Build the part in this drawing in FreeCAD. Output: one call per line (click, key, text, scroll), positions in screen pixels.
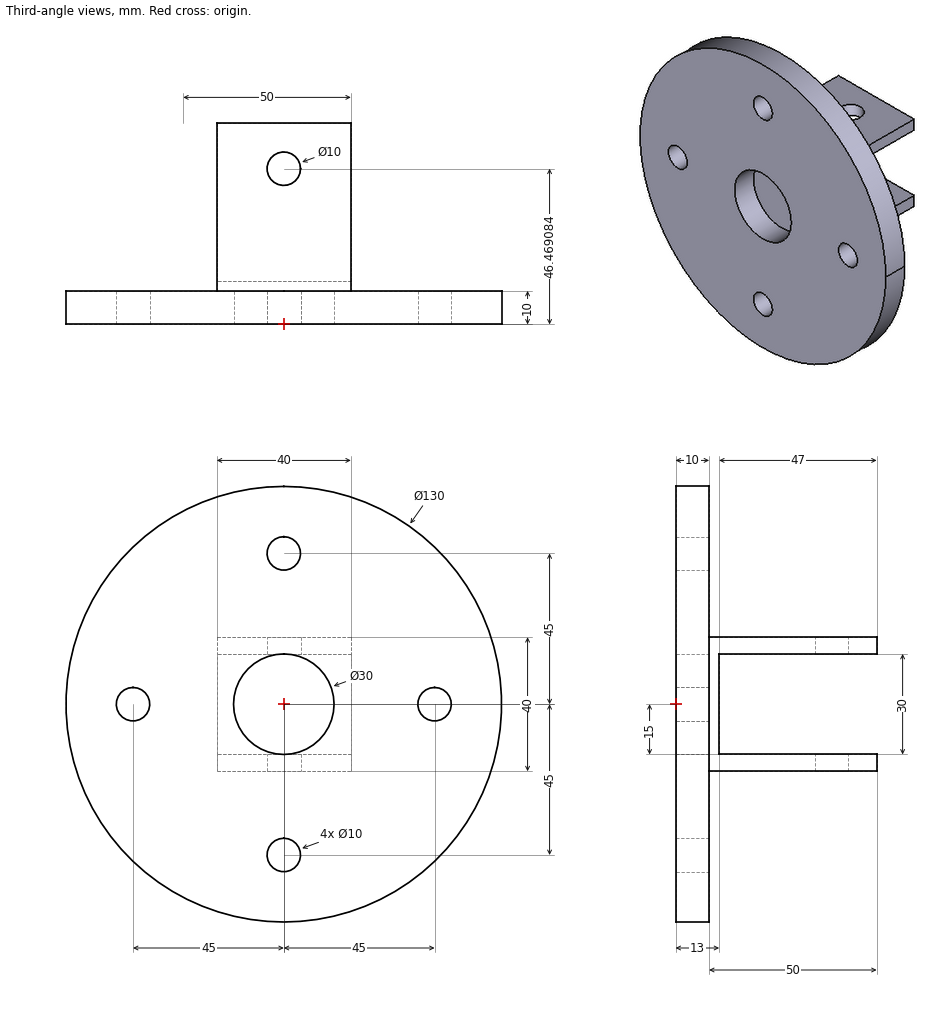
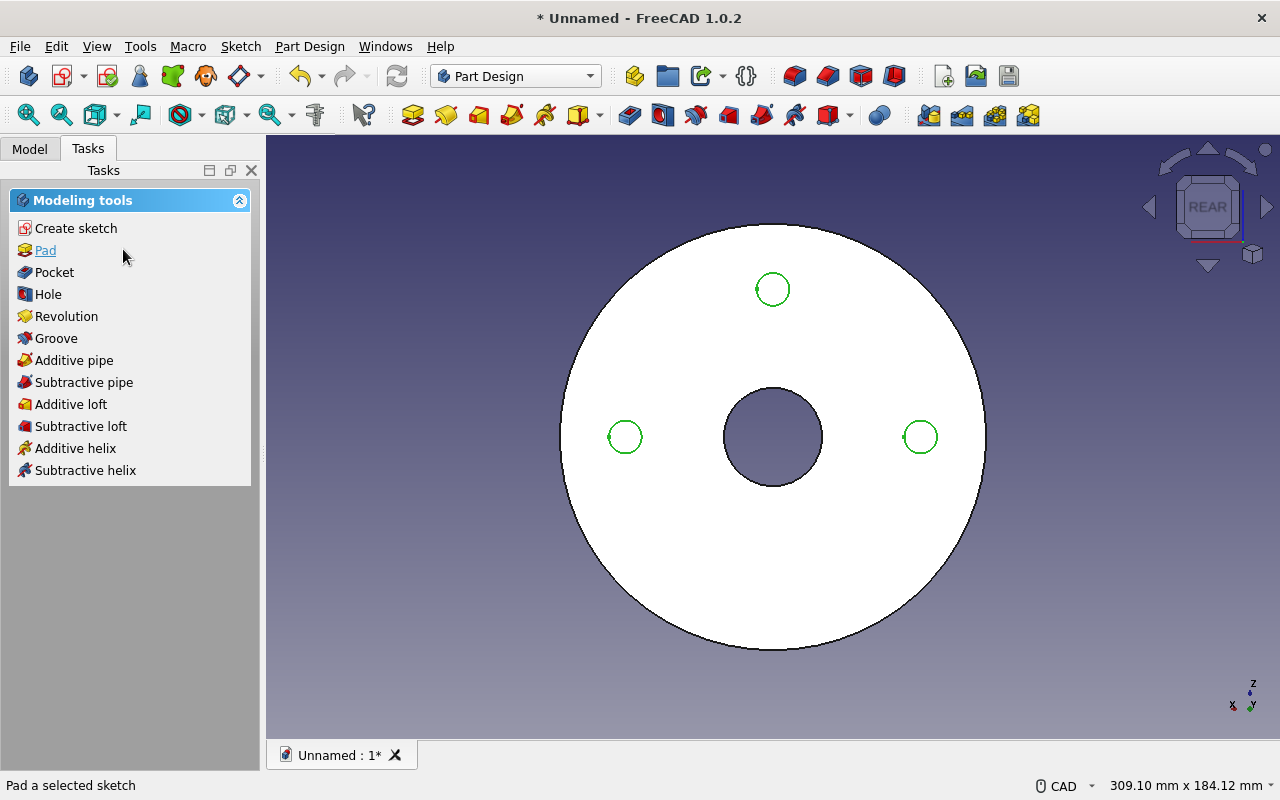
click(630, 116)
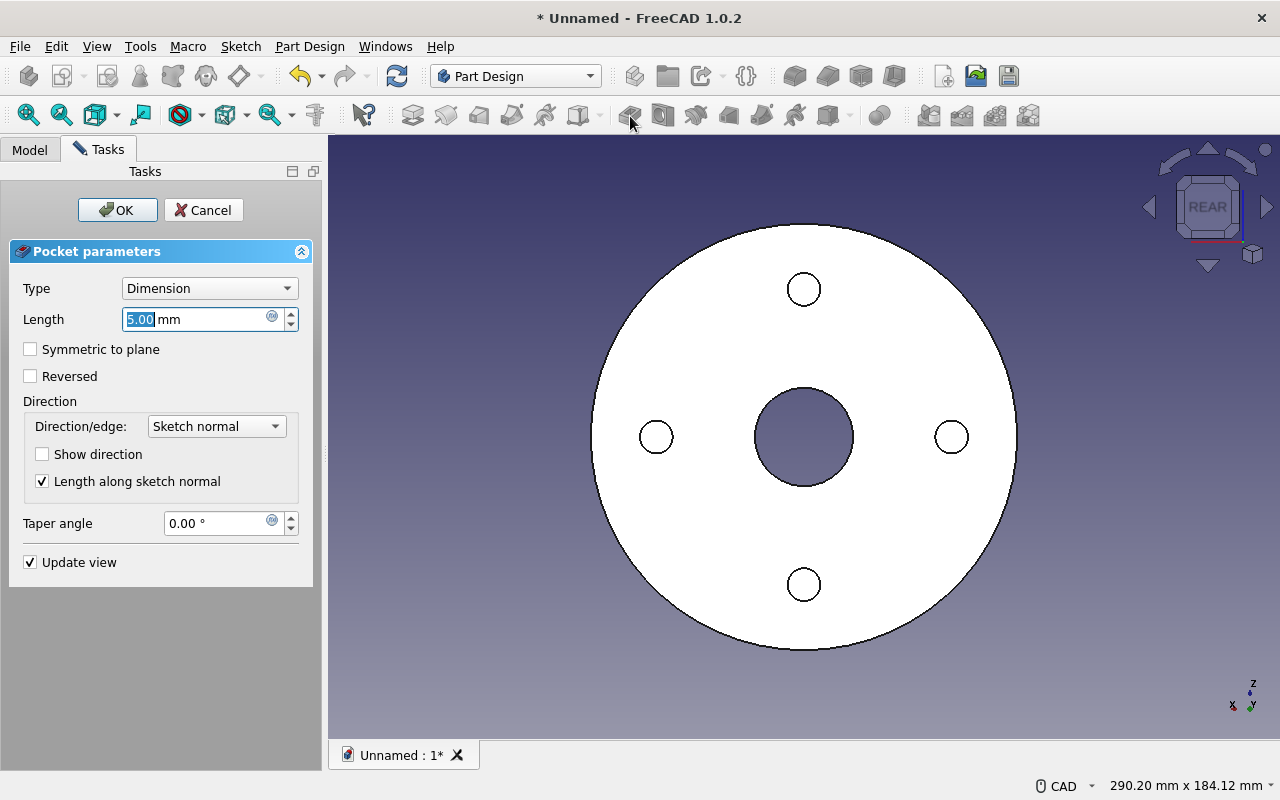
text(10)
key(Tab)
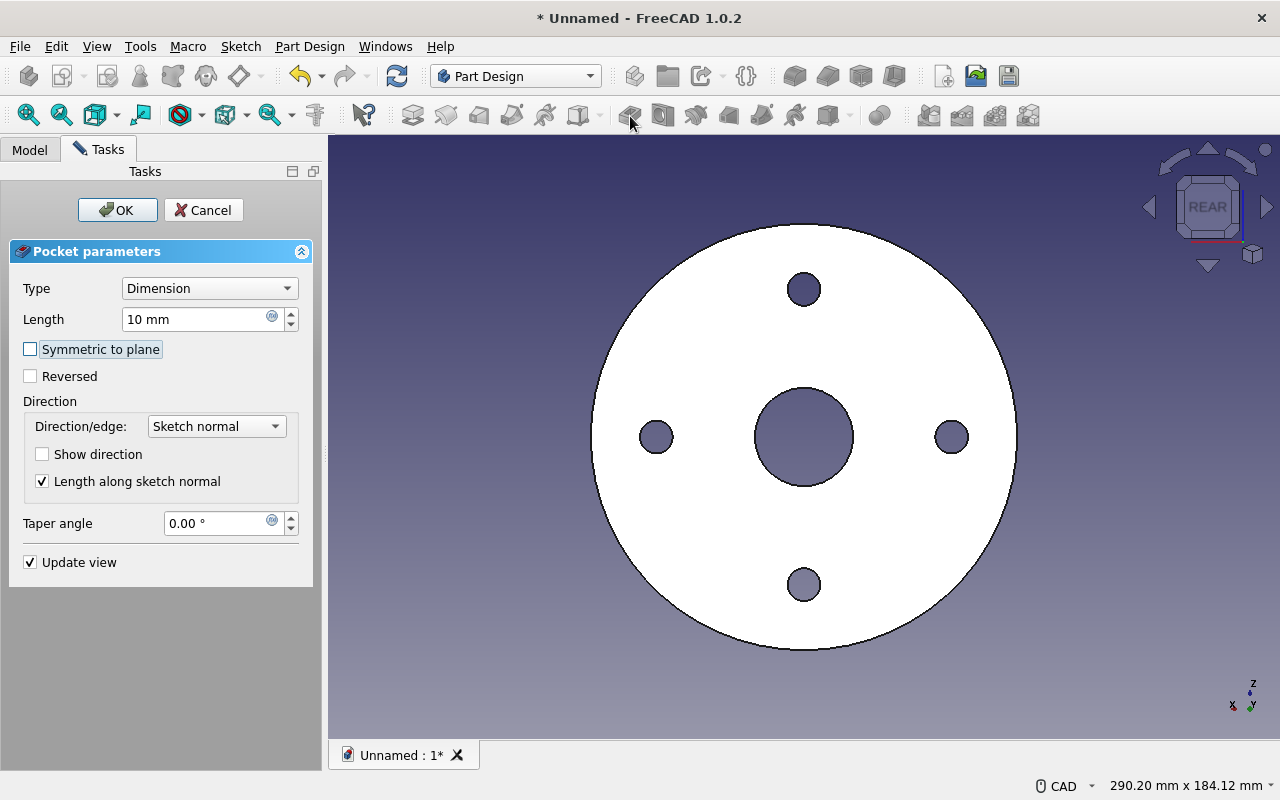
click(118, 210)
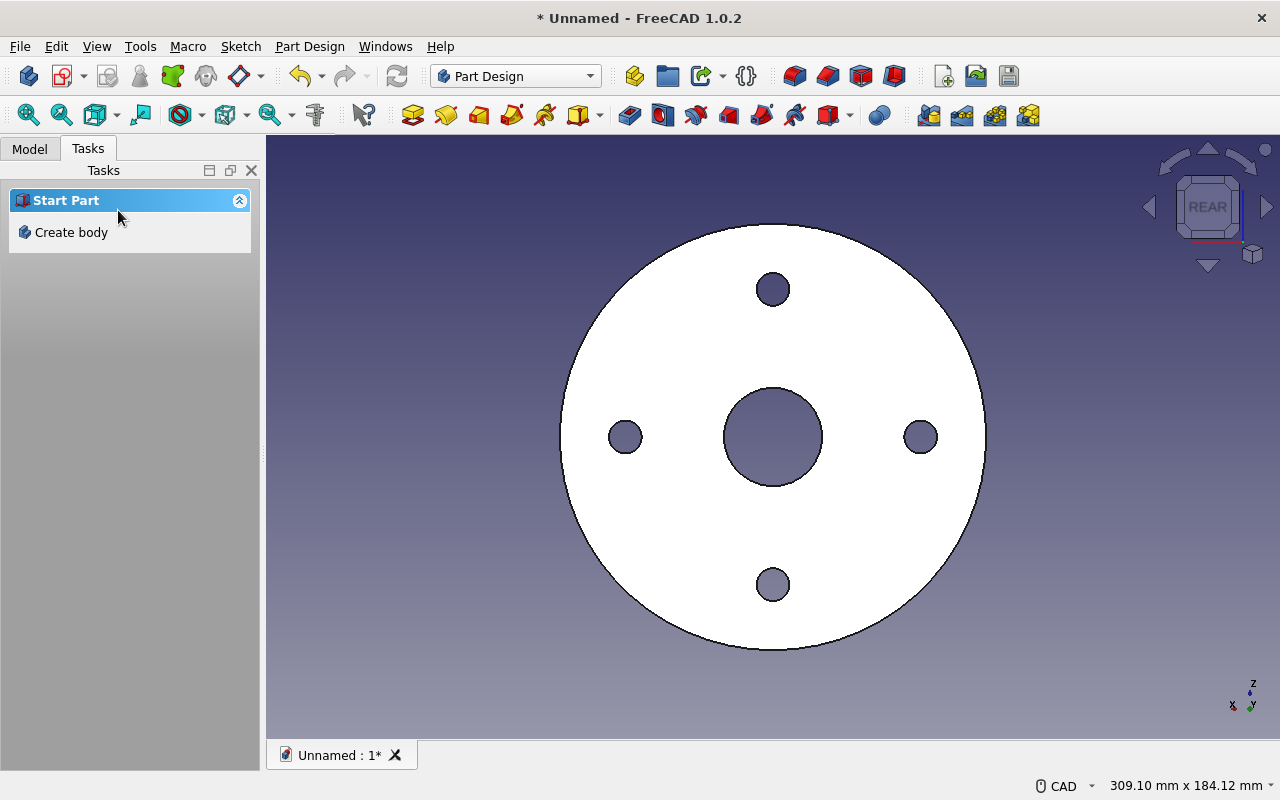
click(834, 314)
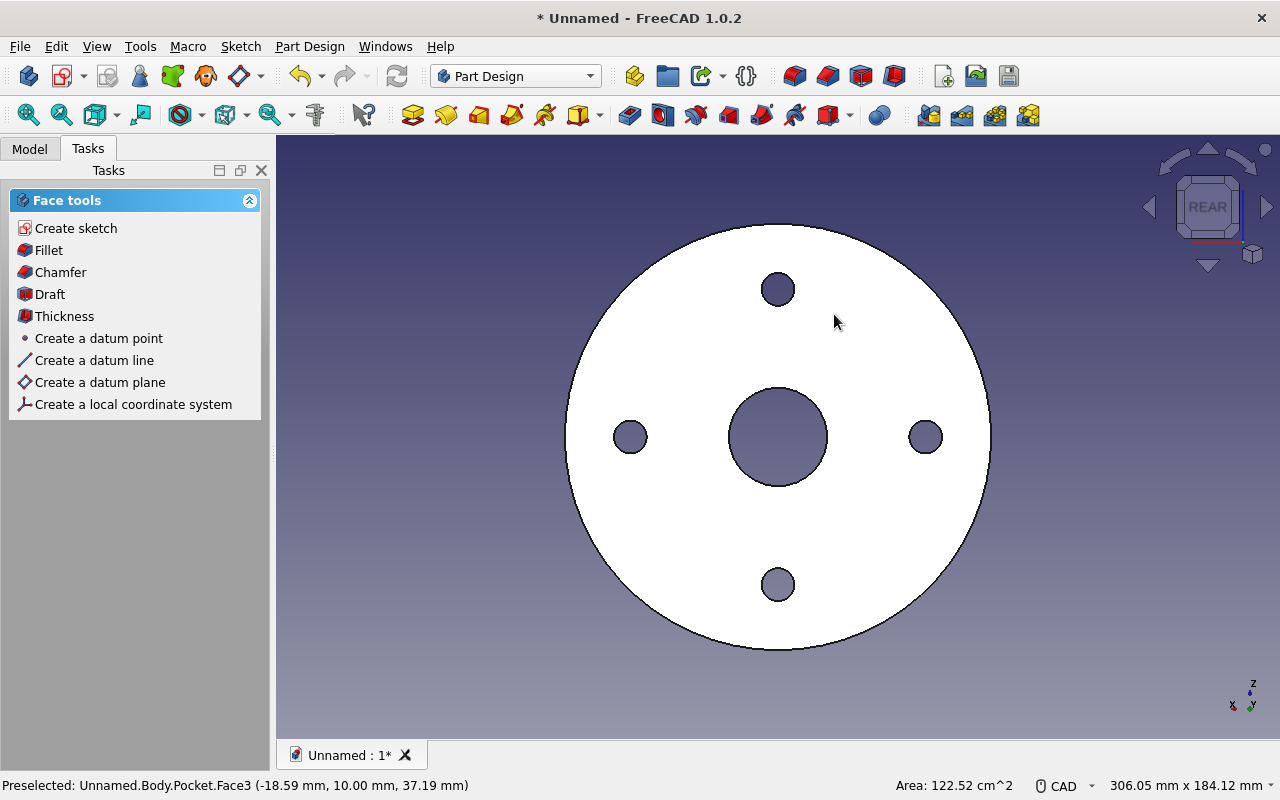
click(62, 76)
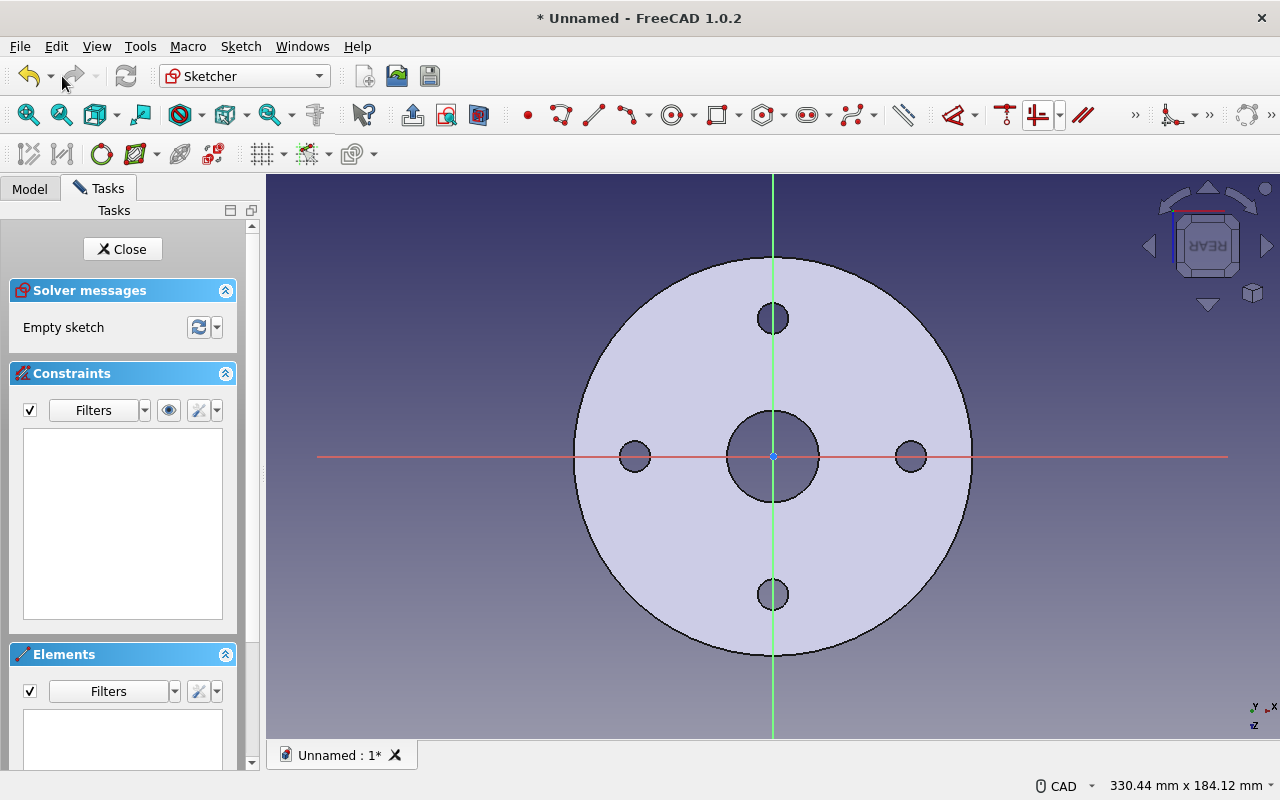
scroll(813, 456, up, 5)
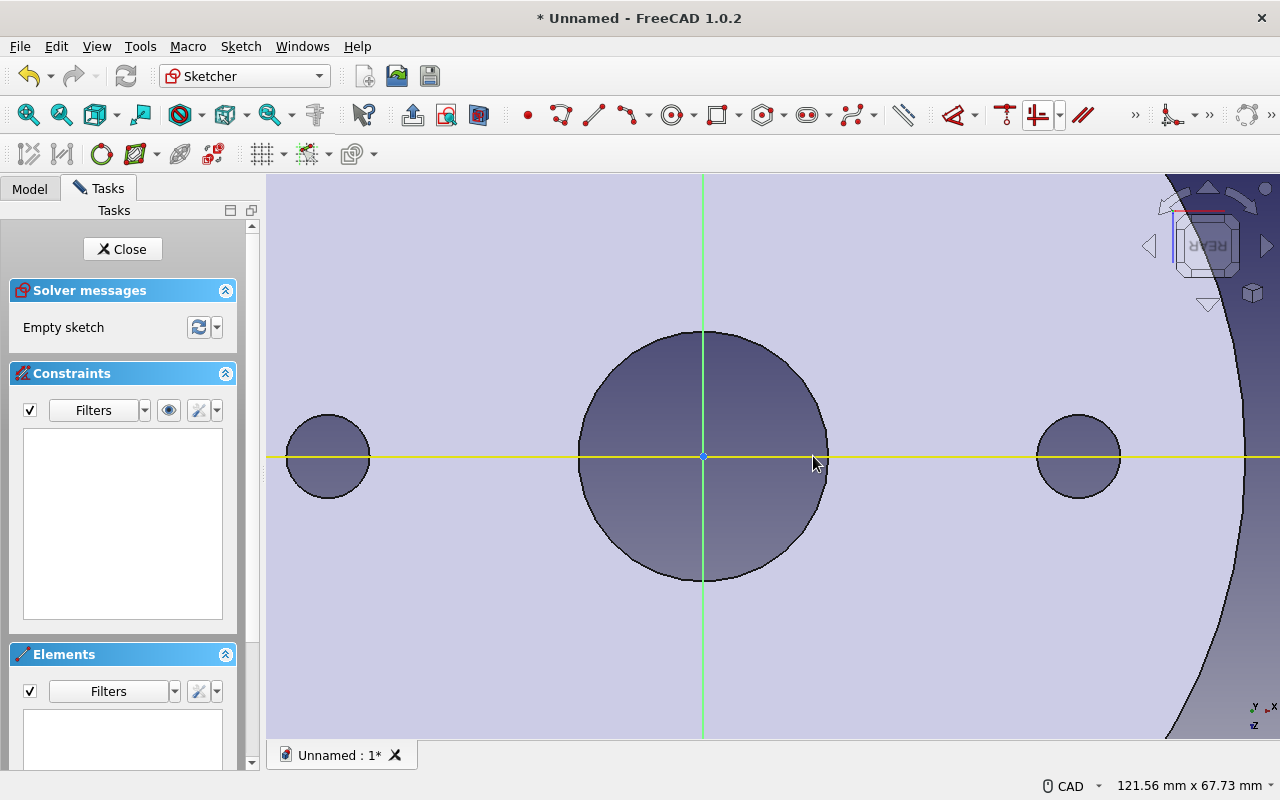
click(738, 116)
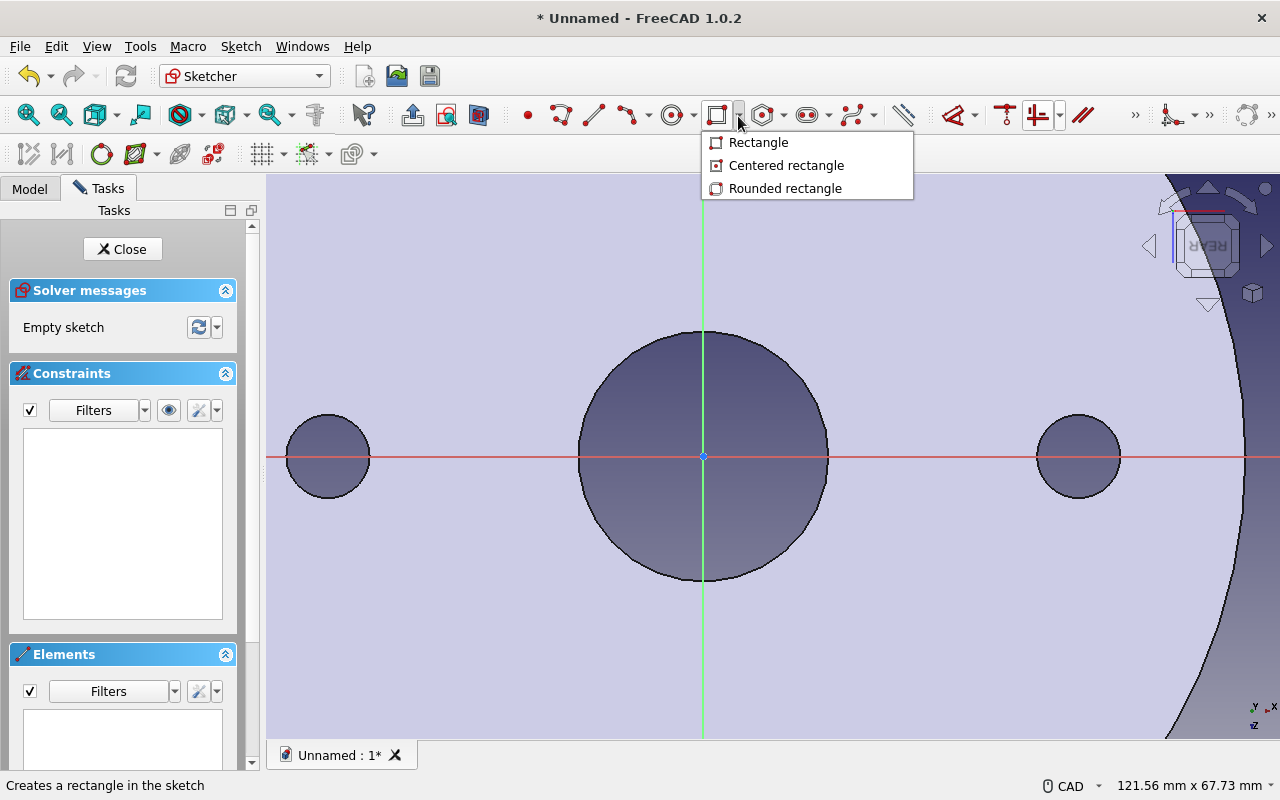
click(808, 166)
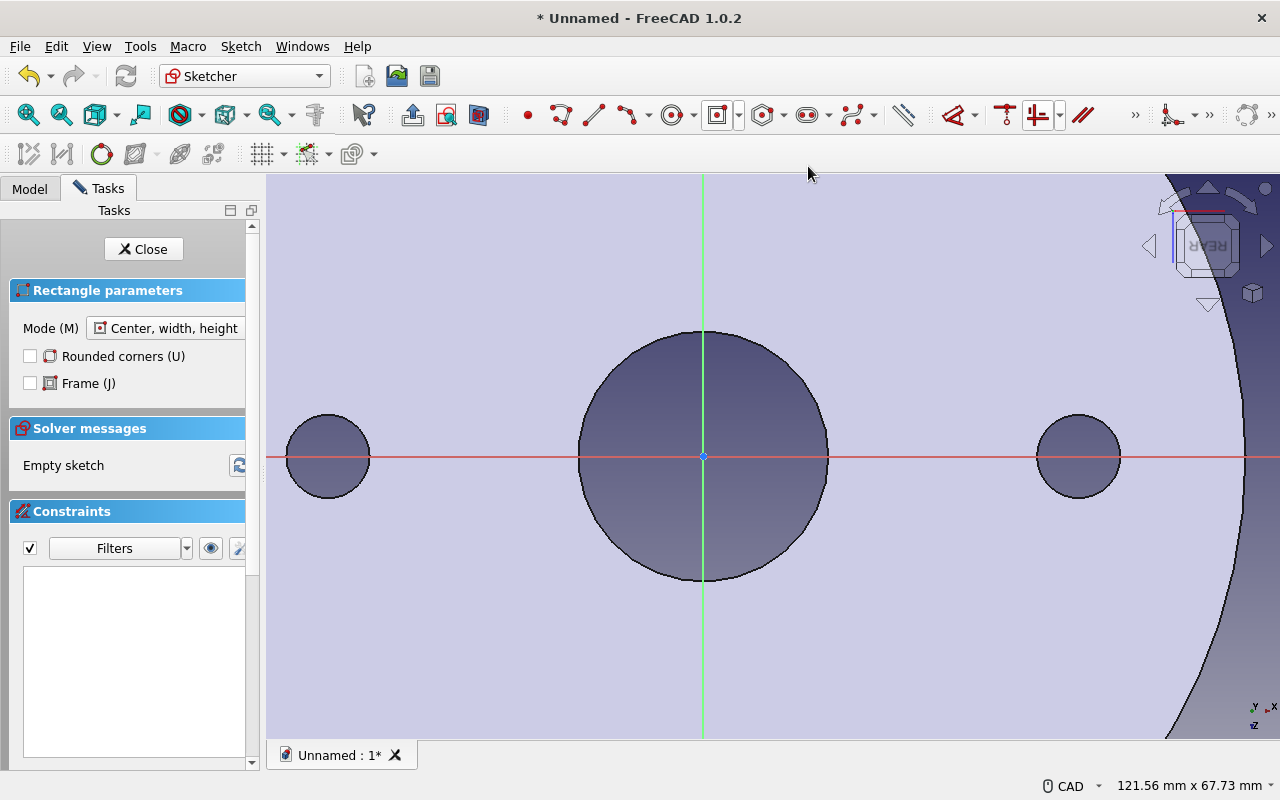
click(703, 456)
move(870, 290)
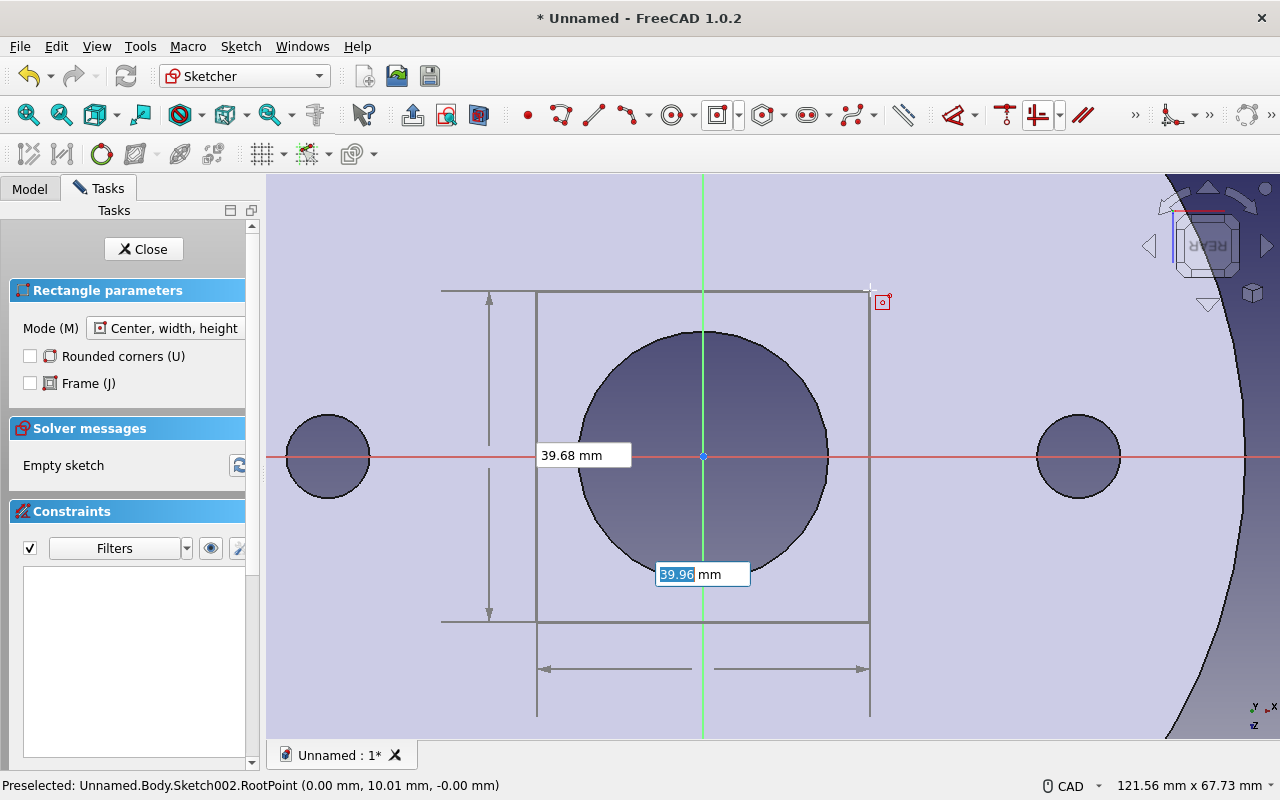
text(40)
key(Tab)
text(40)
key(Return)
key(Escape)